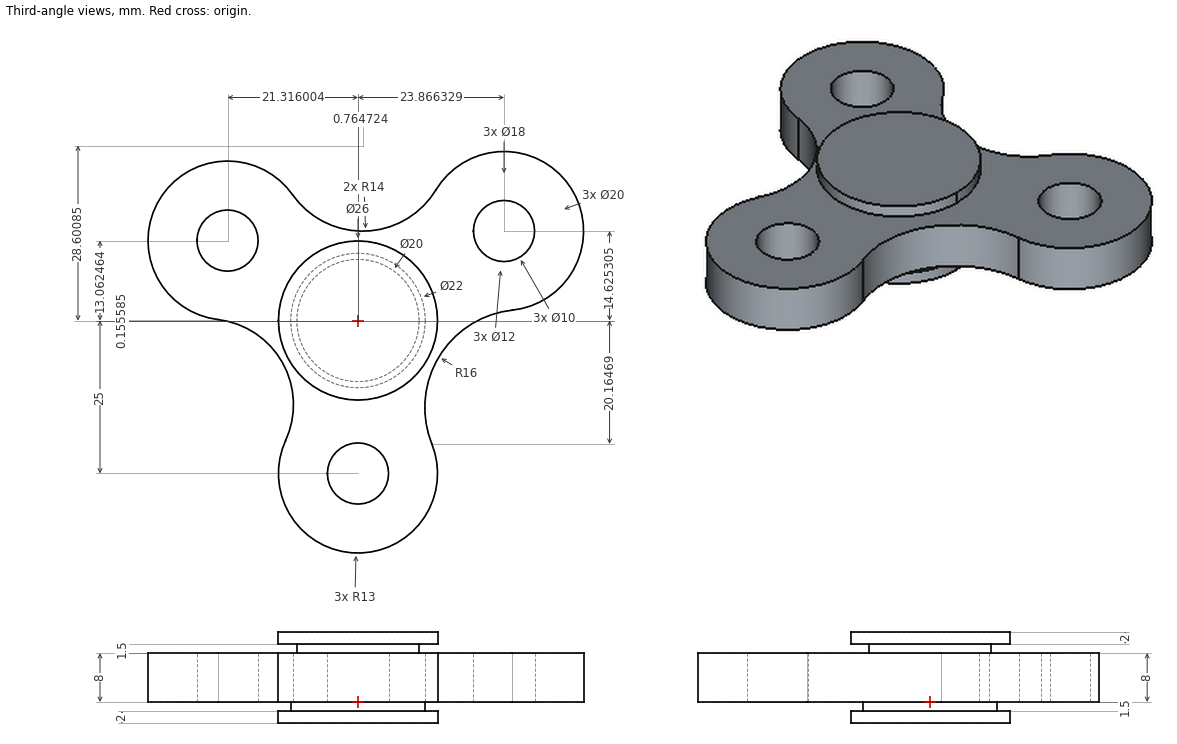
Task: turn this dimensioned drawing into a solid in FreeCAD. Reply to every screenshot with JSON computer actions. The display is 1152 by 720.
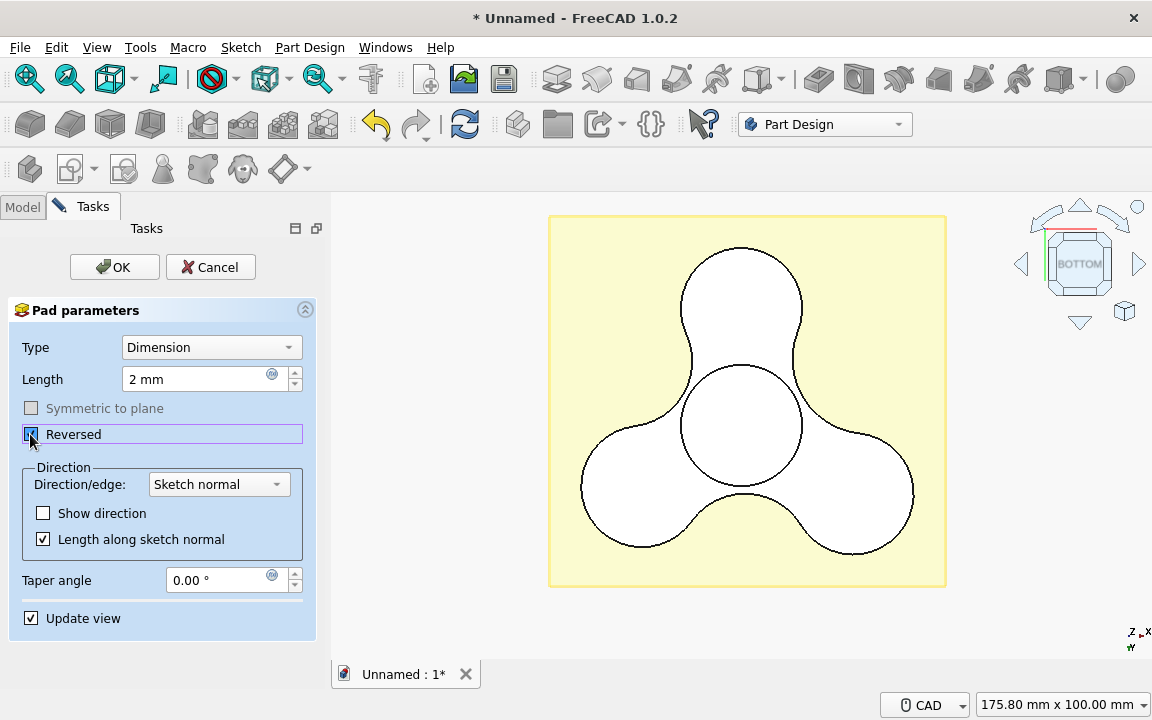
{"action": "left_click", "coordinate": [115, 267]}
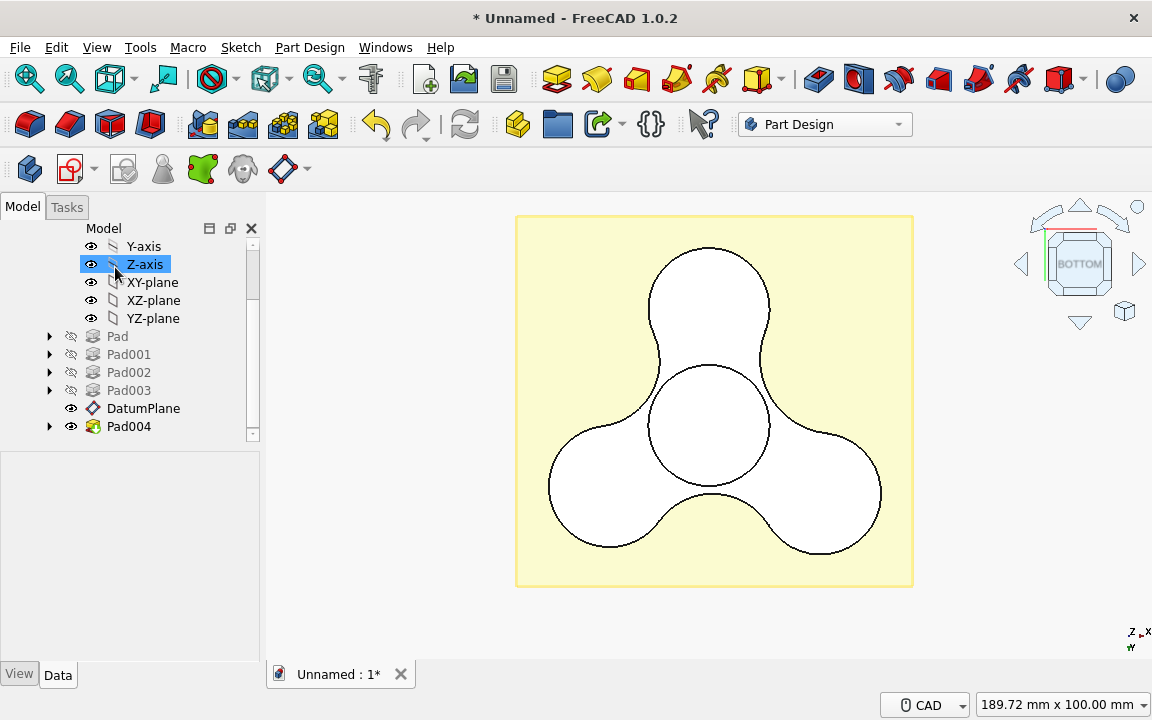
{"action": "left_click", "coordinate": [116, 408]}
{"action": "key", "text": "space"}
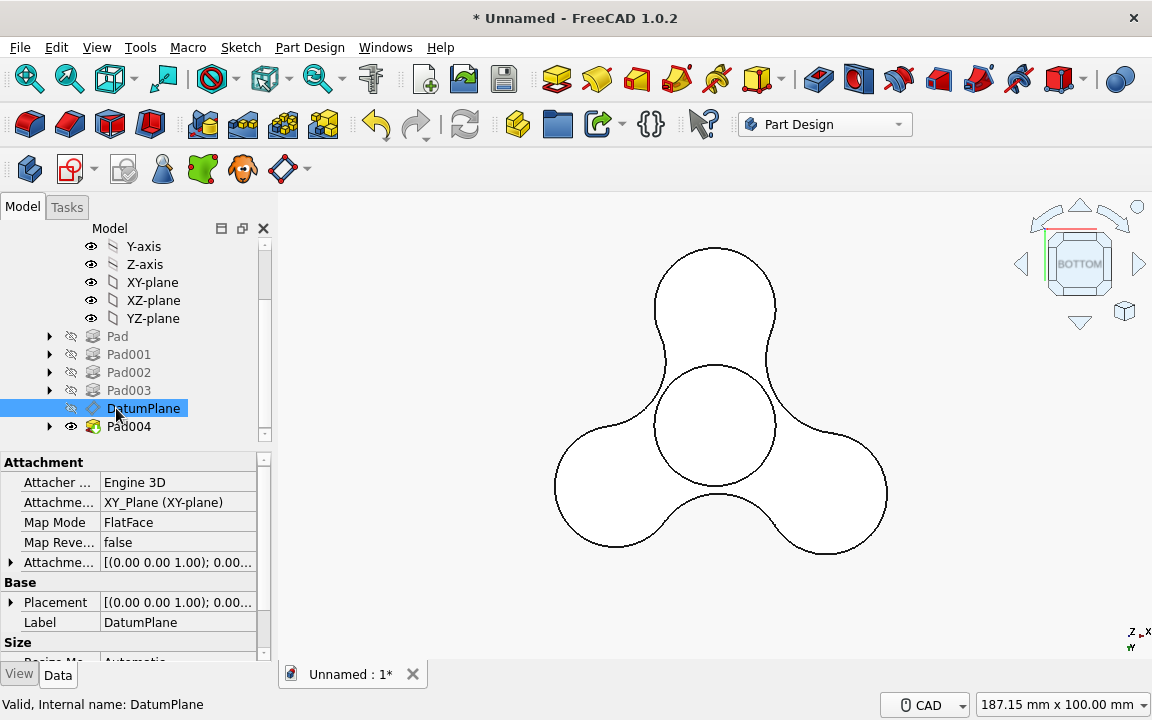
{"action": "left_click", "coordinate": [816, 488]}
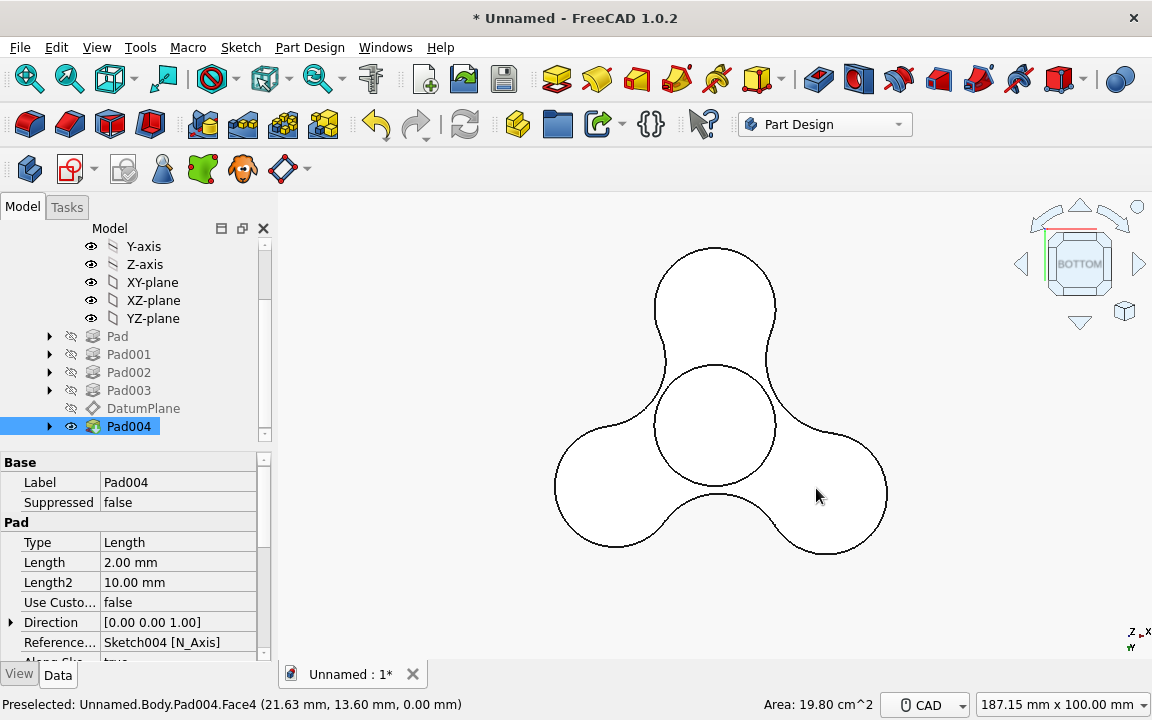
{"action": "left_click", "coordinate": [70, 170]}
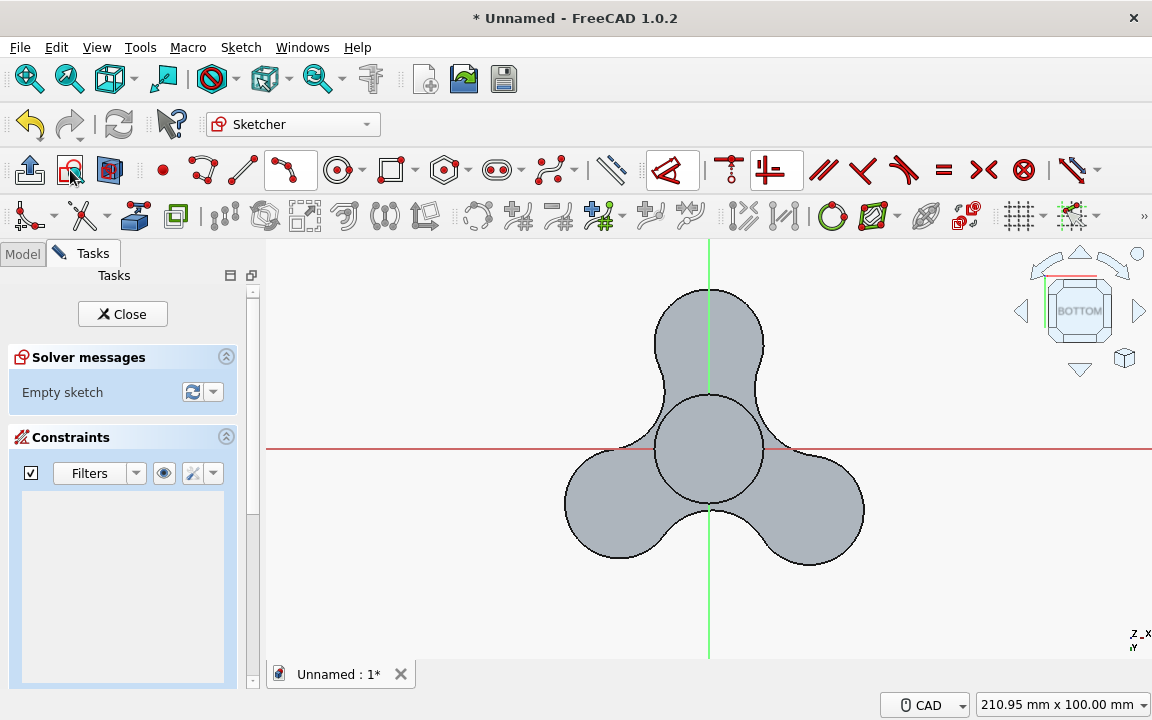
{"action": "left_click", "coordinate": [338, 170]}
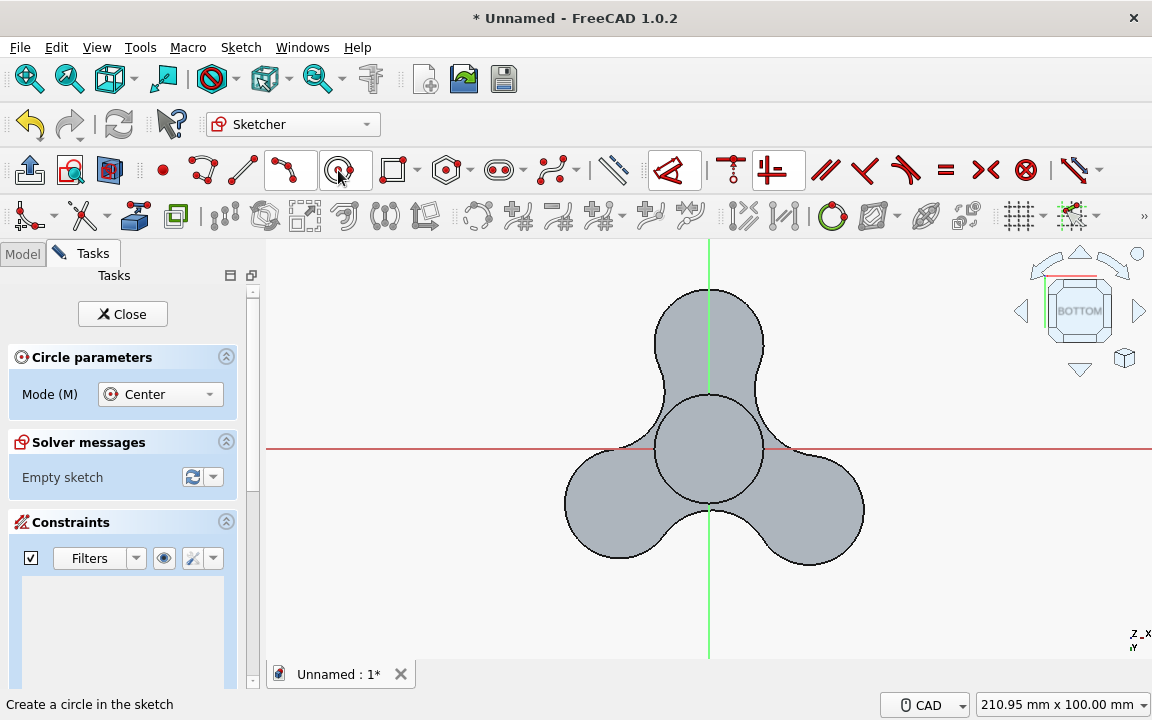
{"action": "left_click", "coordinate": [809, 510]}
{"action": "mouse_move", "coordinate": [839, 481]}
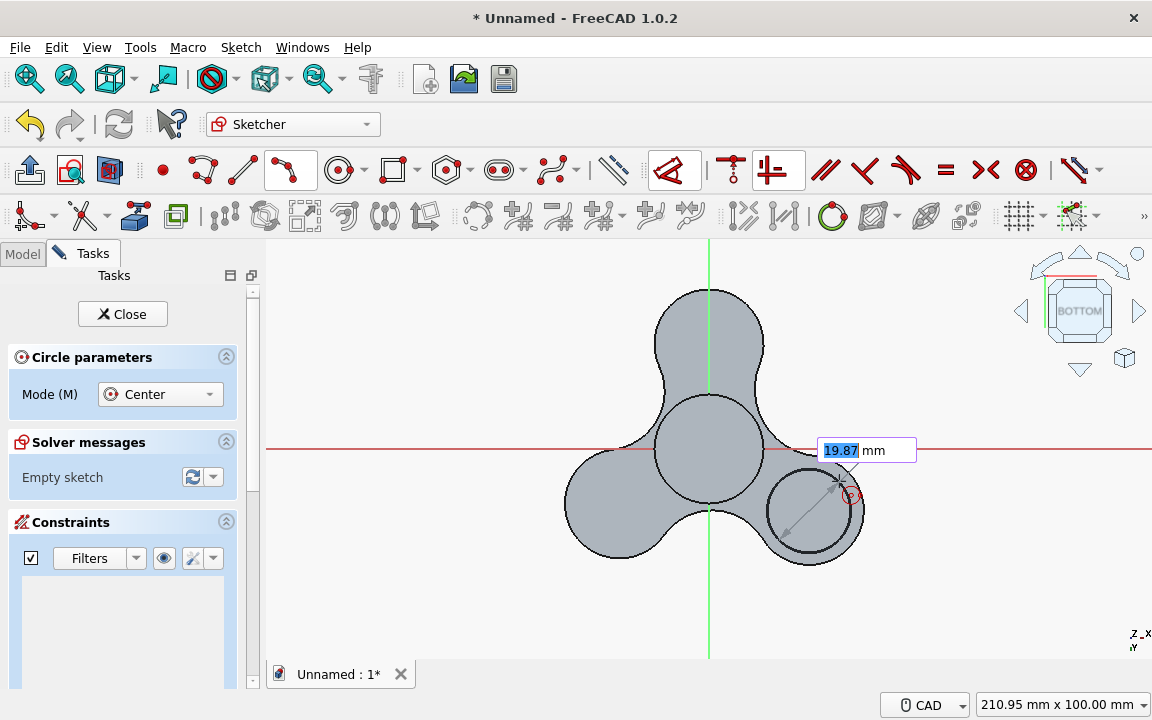
{"action": "type", "text": "20"}
{"action": "key", "text": "Return"}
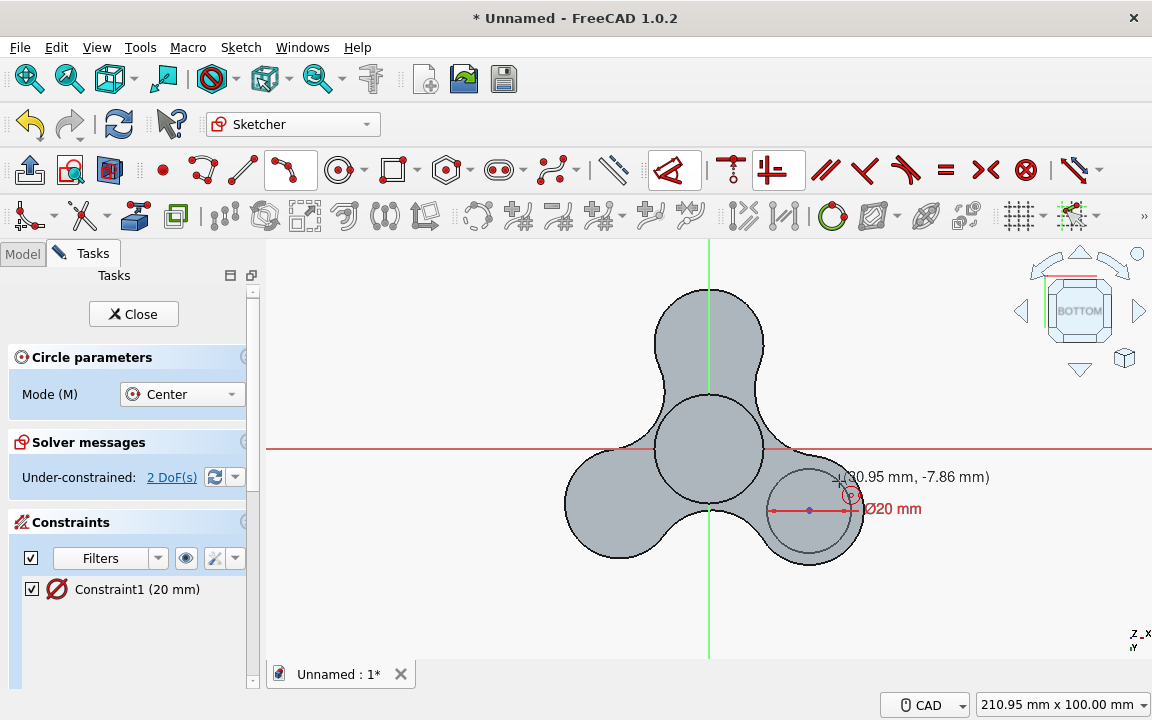
{"action": "left_click", "coordinate": [619, 504]}
{"action": "mouse_move", "coordinate": [649, 474]}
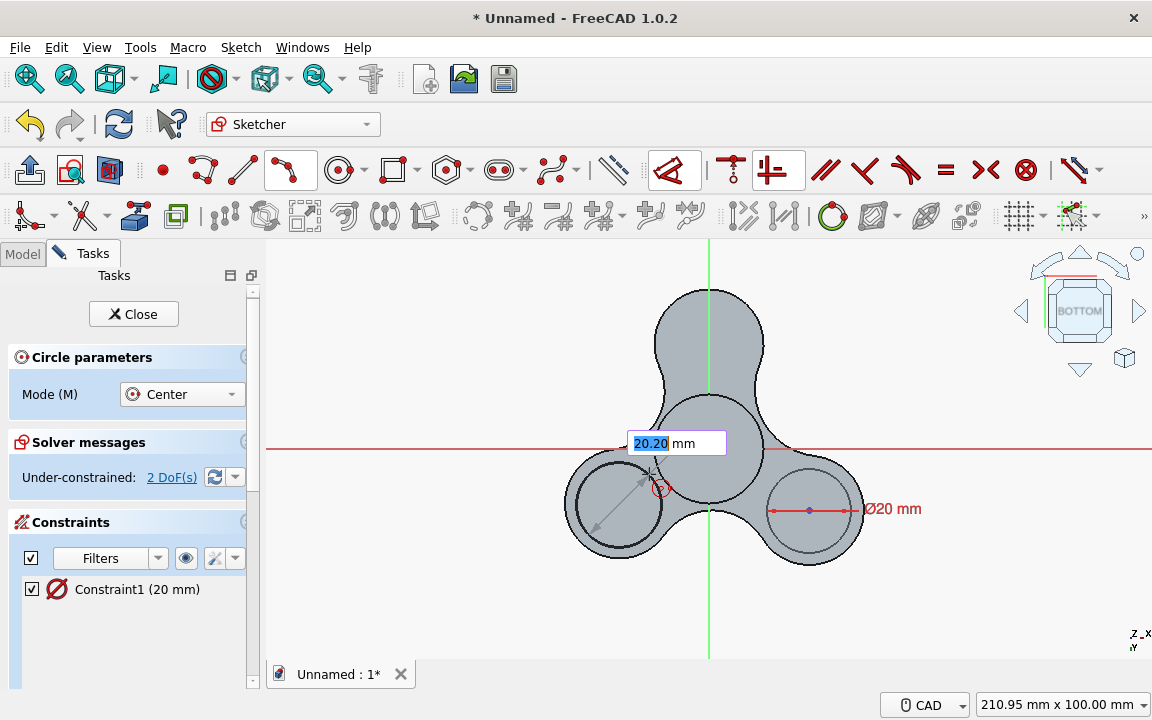
{"action": "type", "text": "20"}
{"action": "key", "text": "Return"}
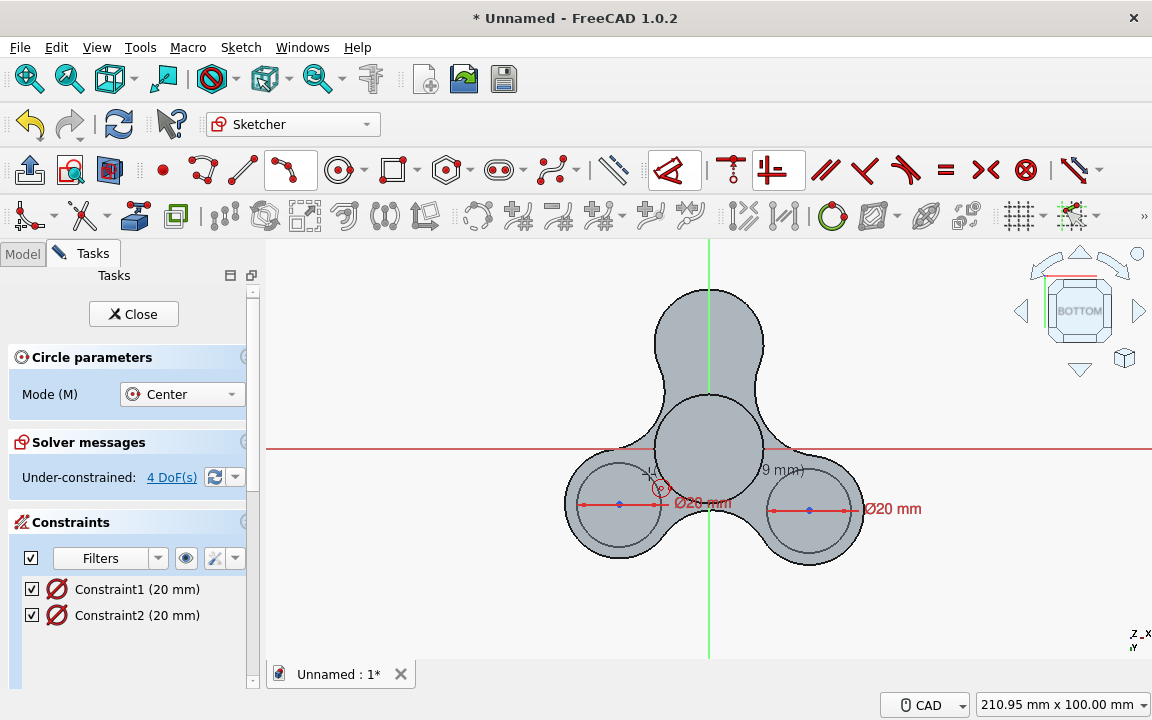
{"action": "left_click", "coordinate": [709, 344]}
{"action": "mouse_move", "coordinate": [739, 314]}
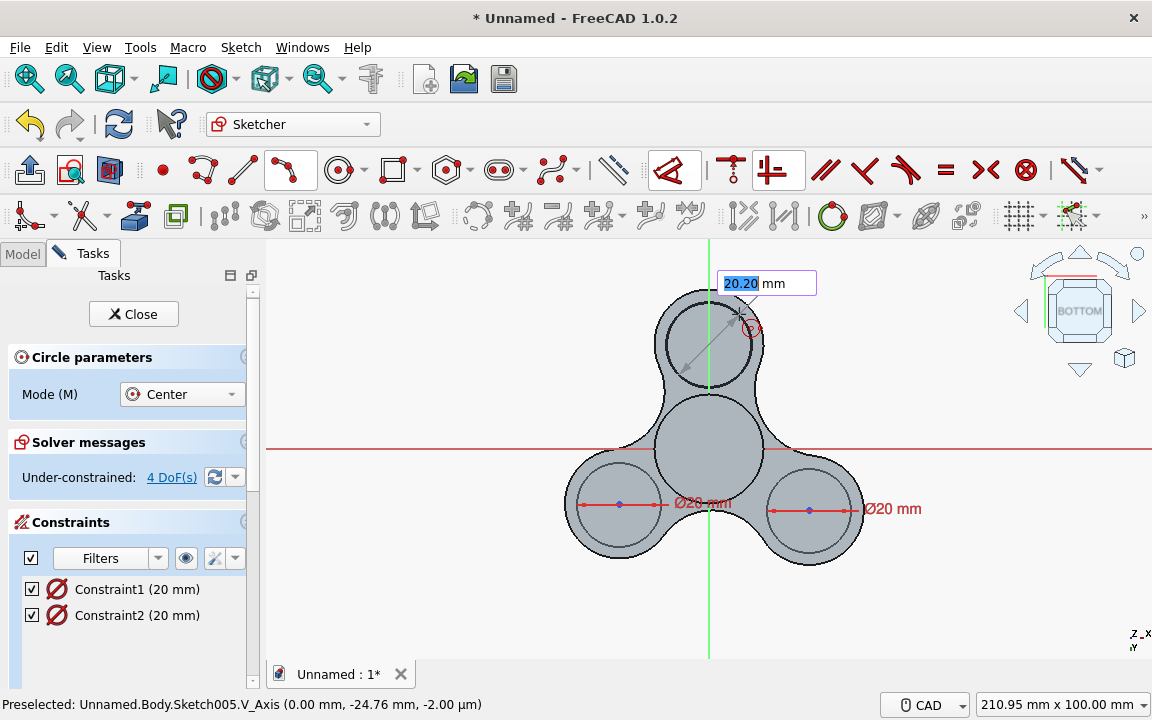
{"action": "type", "text": "20"}
{"action": "key", "text": "Return"}
{"action": "key", "text": "Escape"}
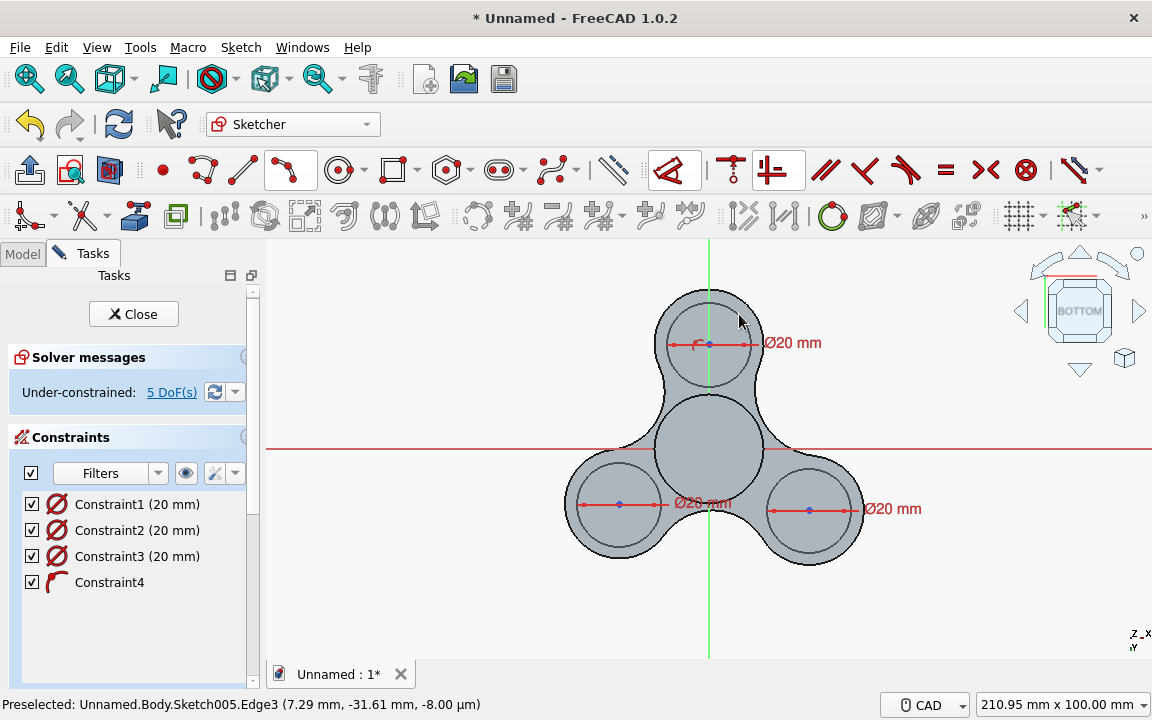
{"action": "left_click", "coordinate": [709, 345]}